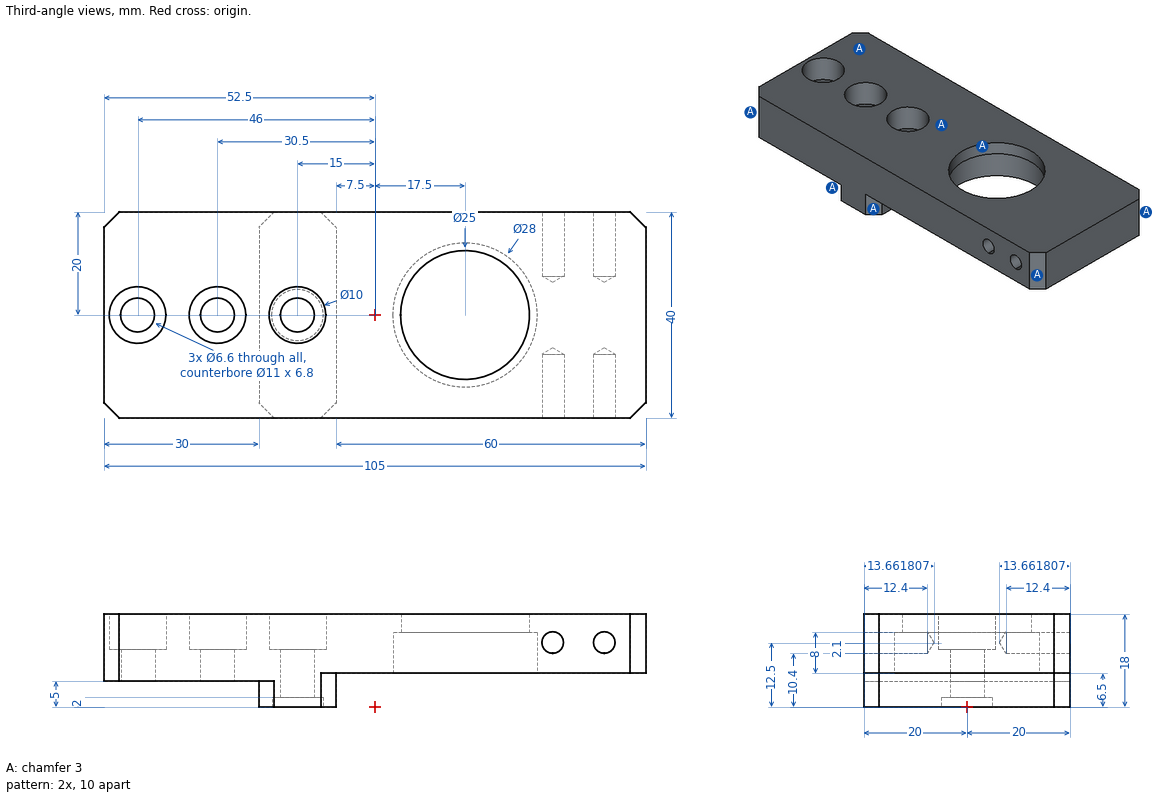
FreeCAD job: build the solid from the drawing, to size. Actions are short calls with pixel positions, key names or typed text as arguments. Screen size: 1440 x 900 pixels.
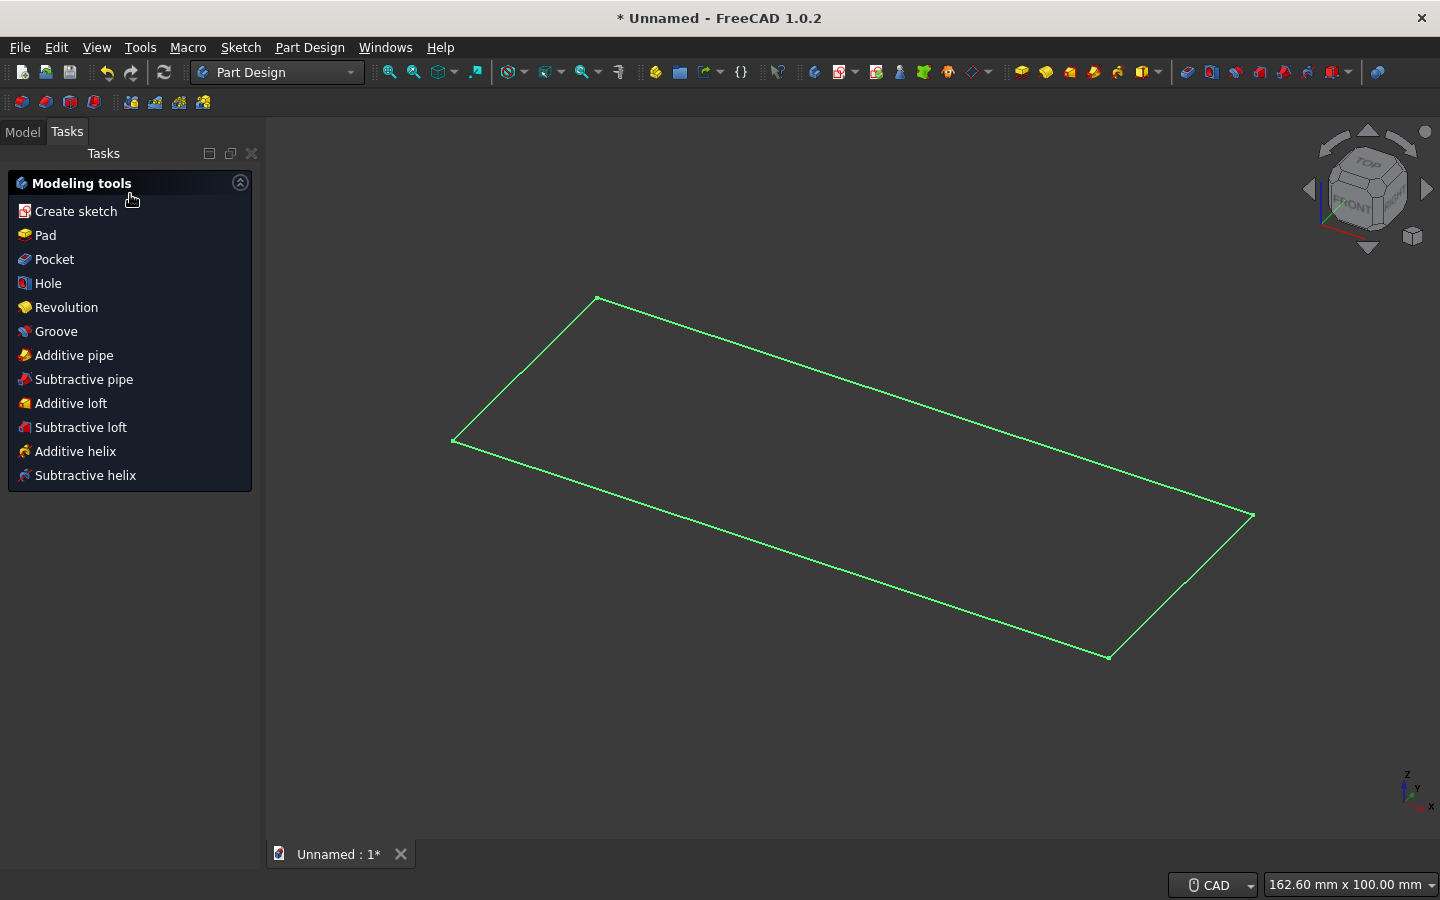
click(1022, 72)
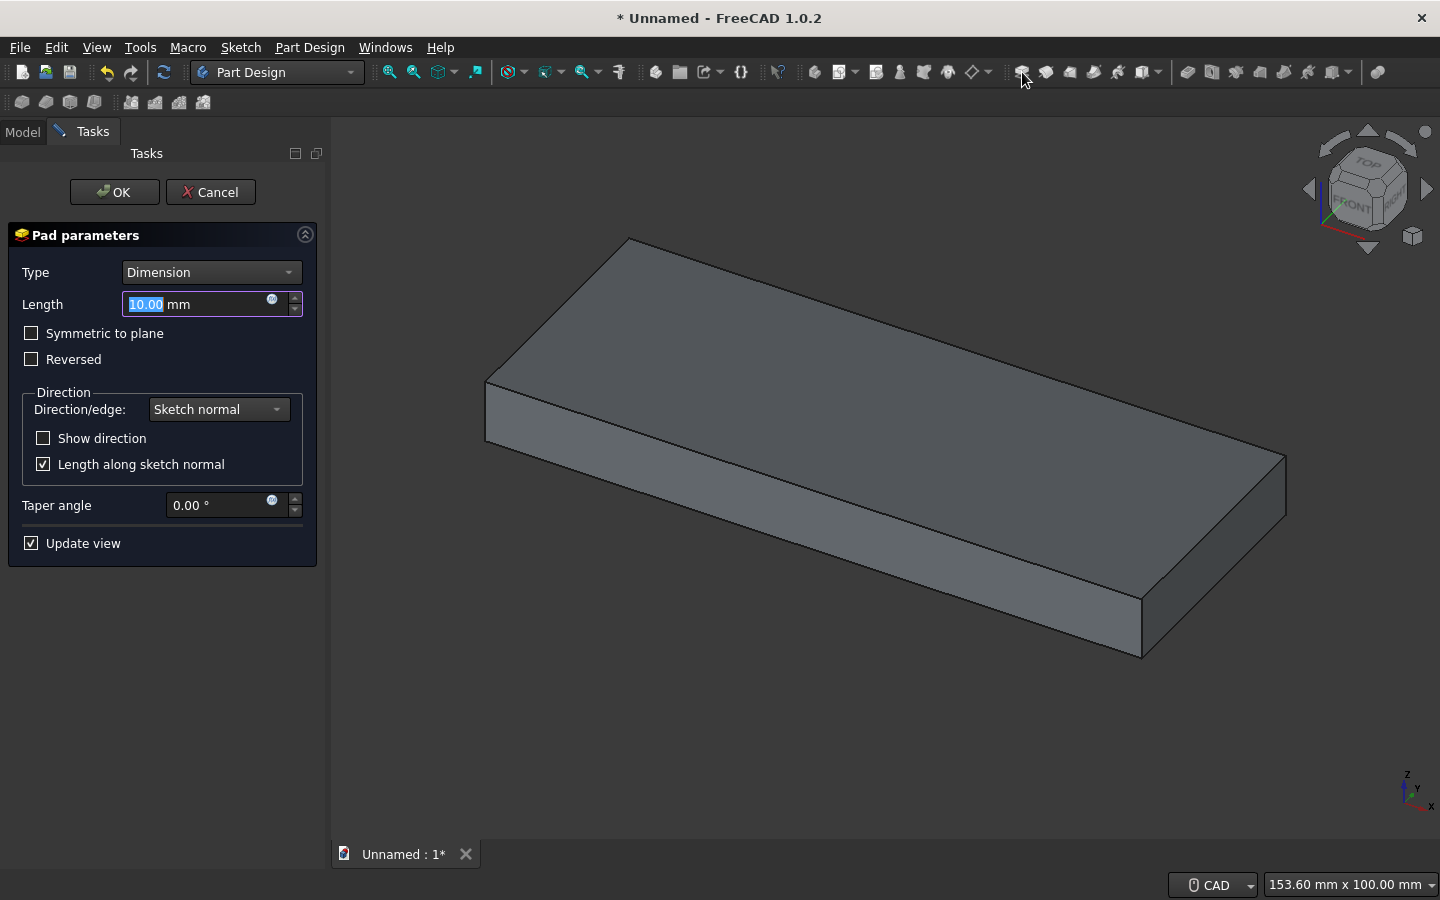
text(18)
key(Tab)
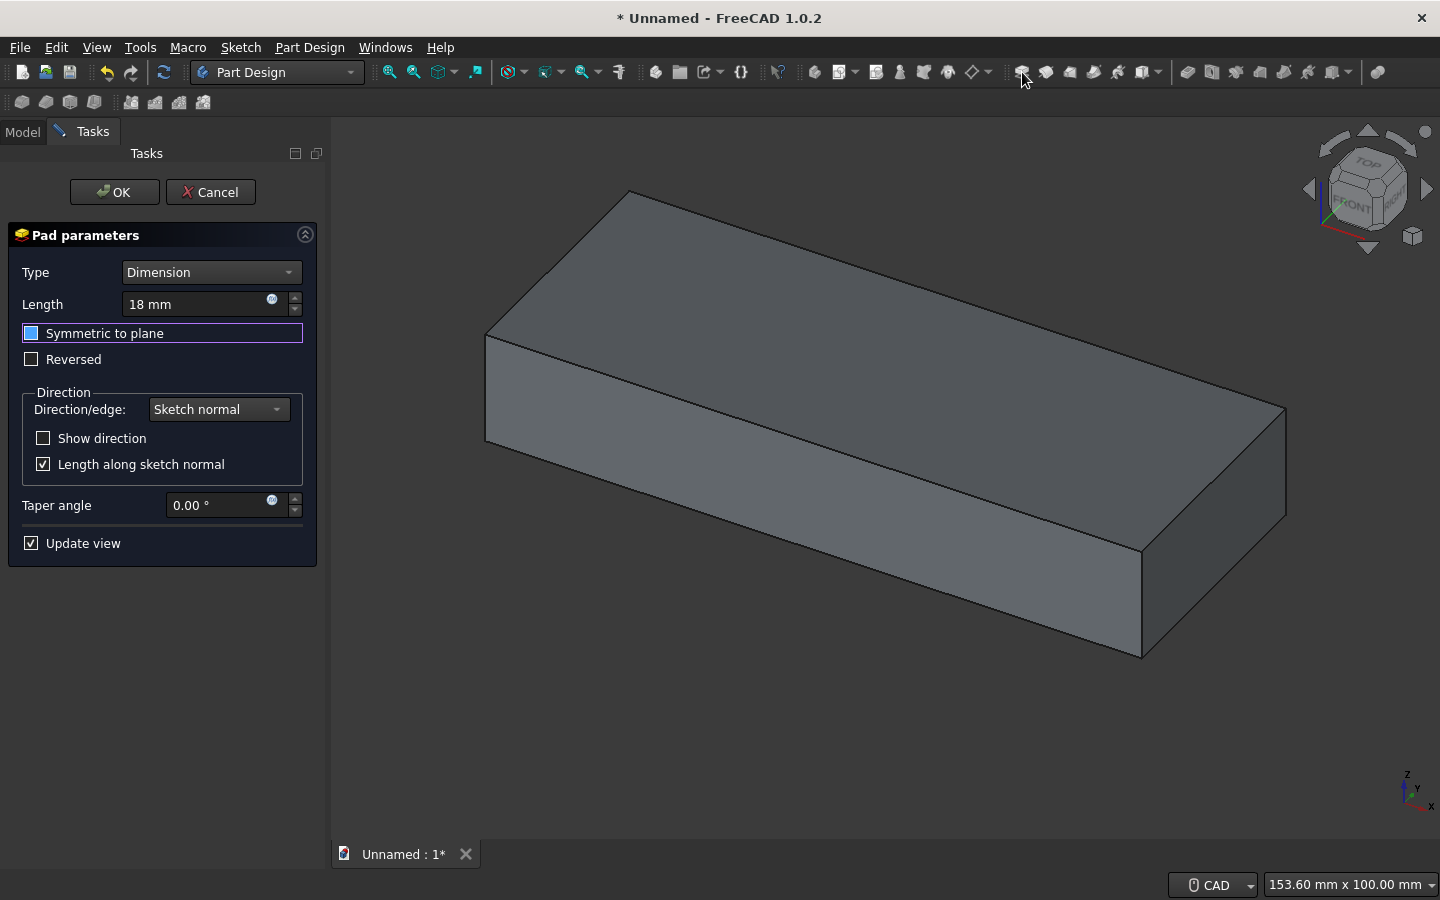
click(115, 192)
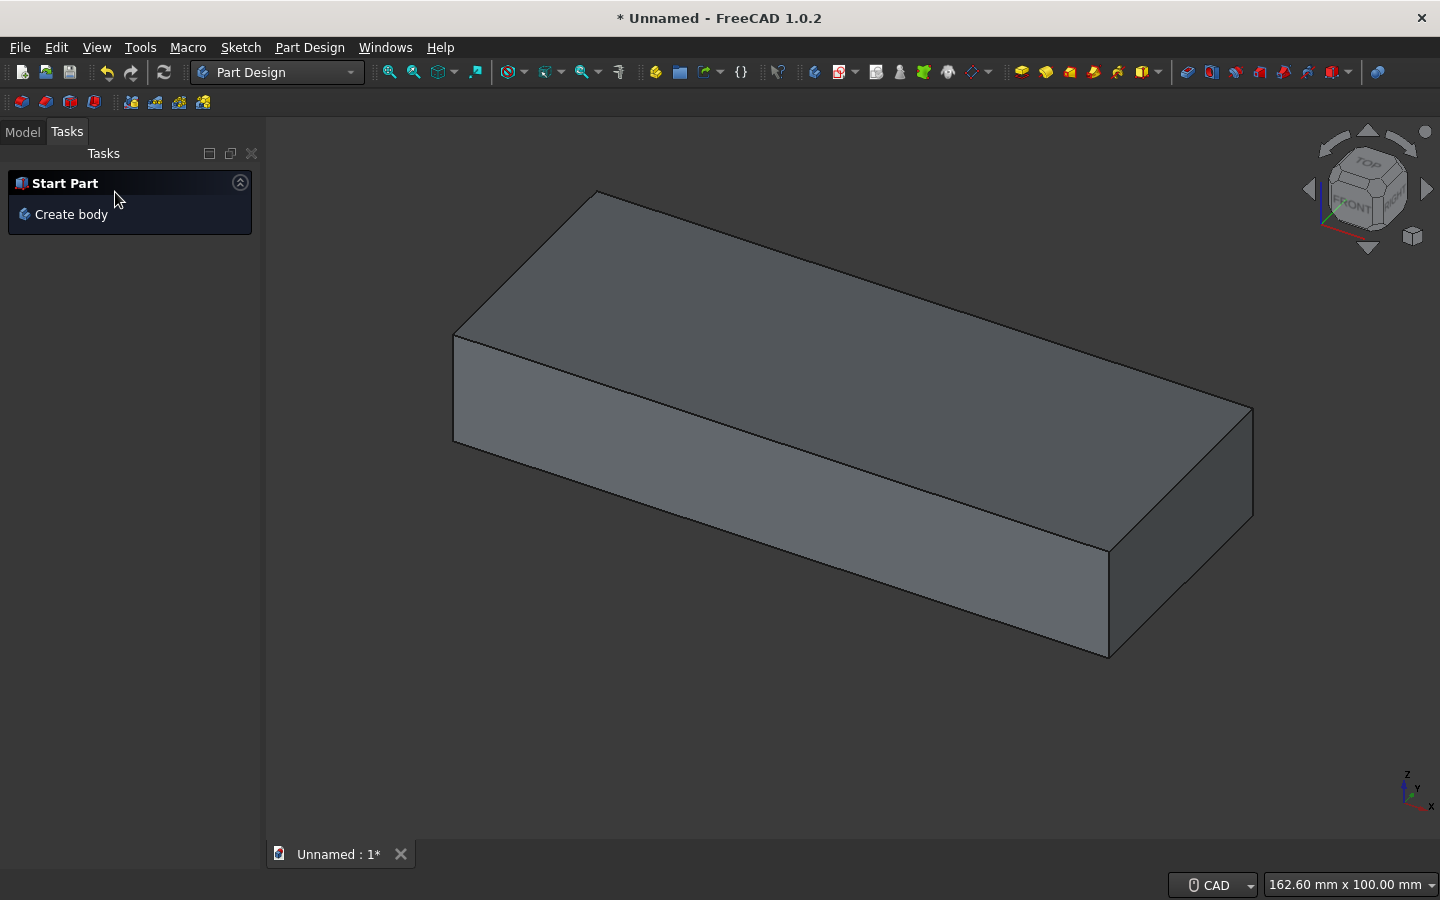
click(840, 72)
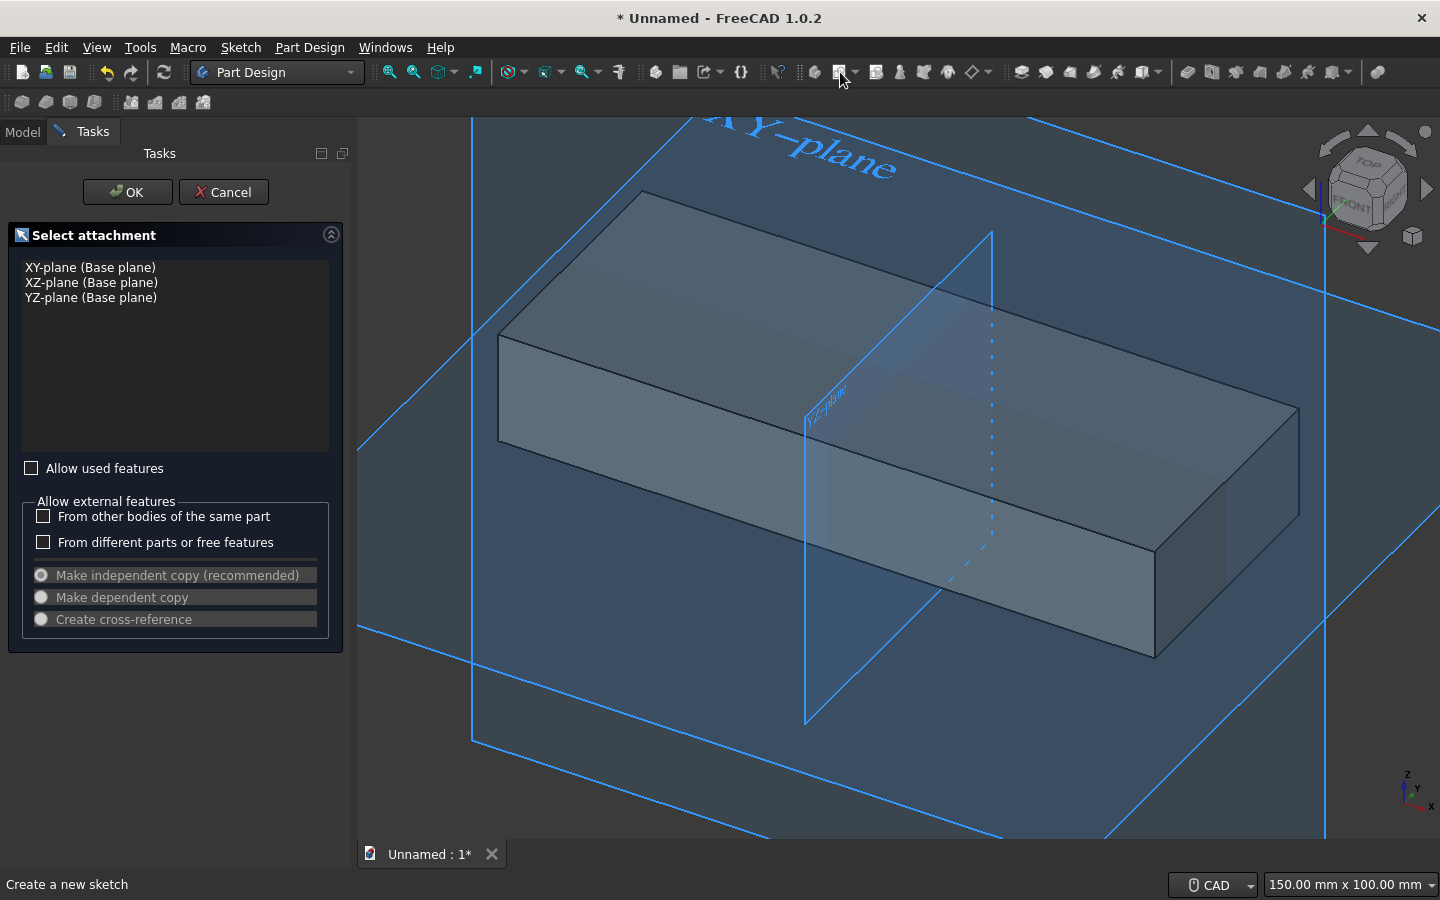
click(82, 268)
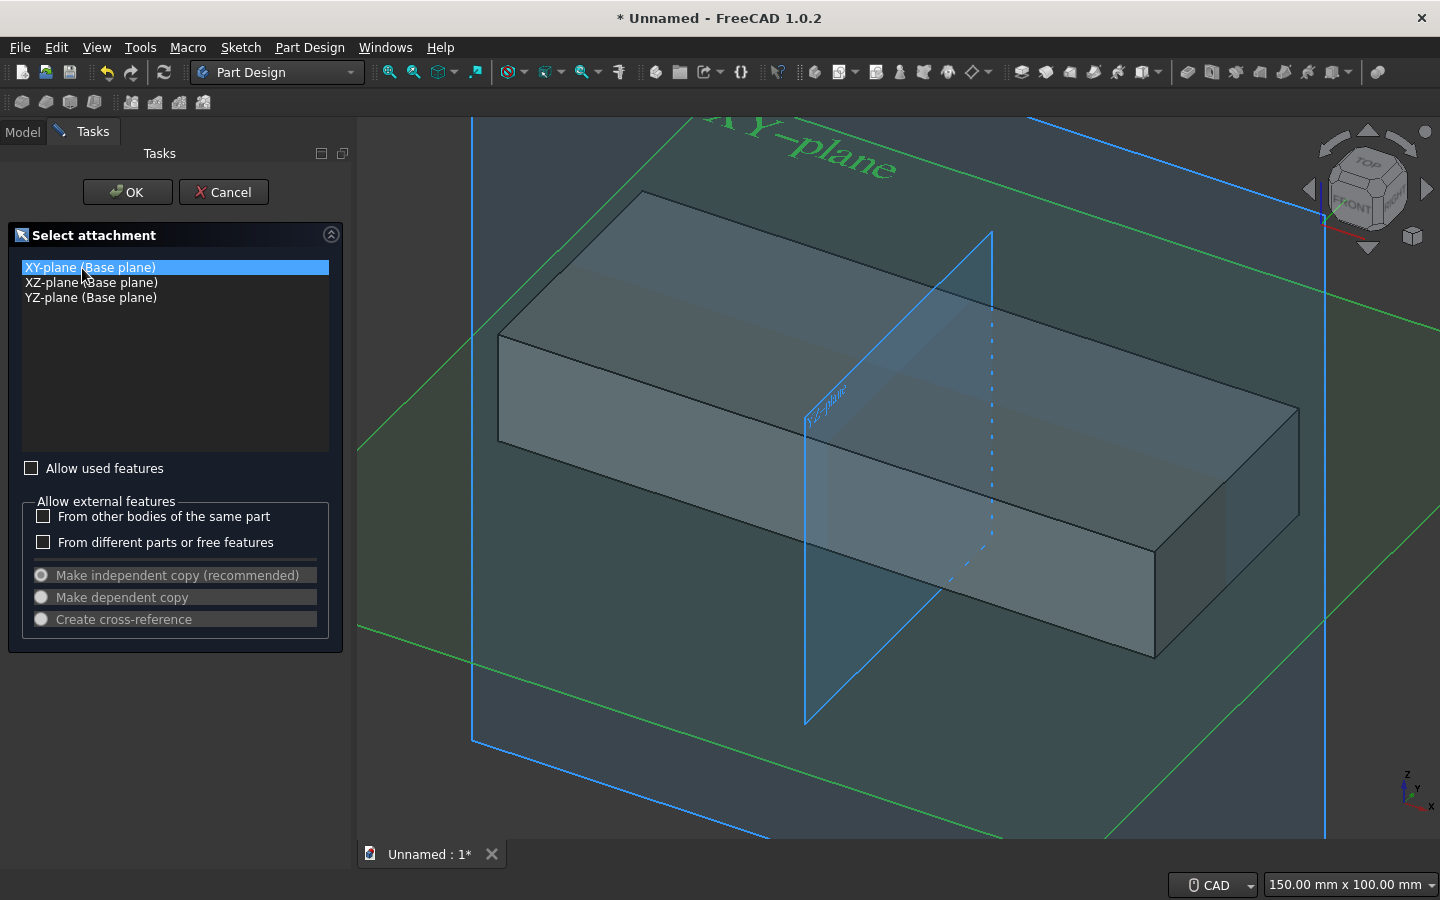
click(128, 192)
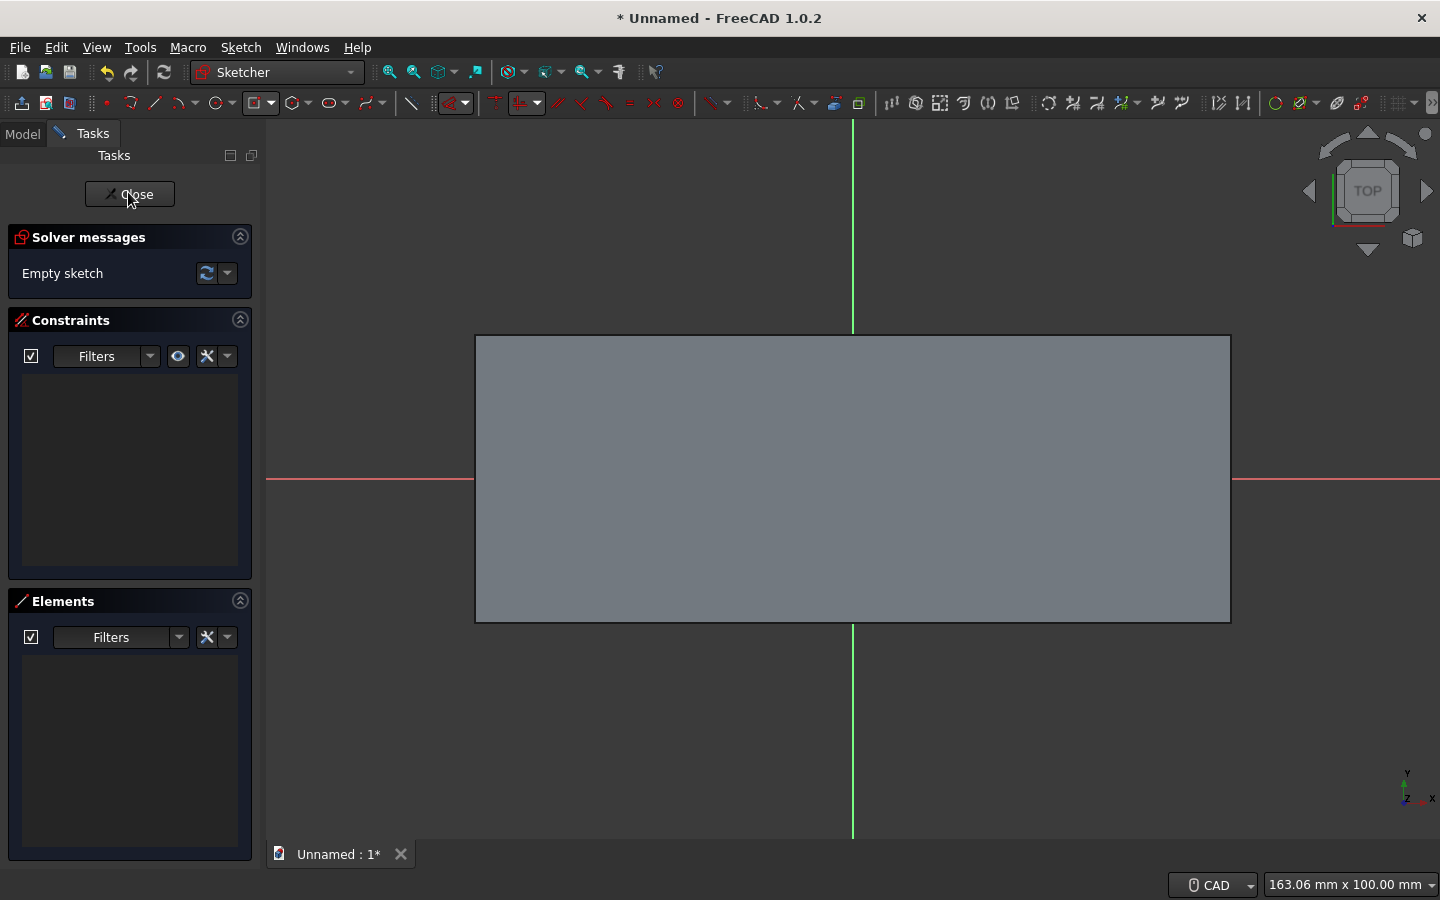
click(70, 104)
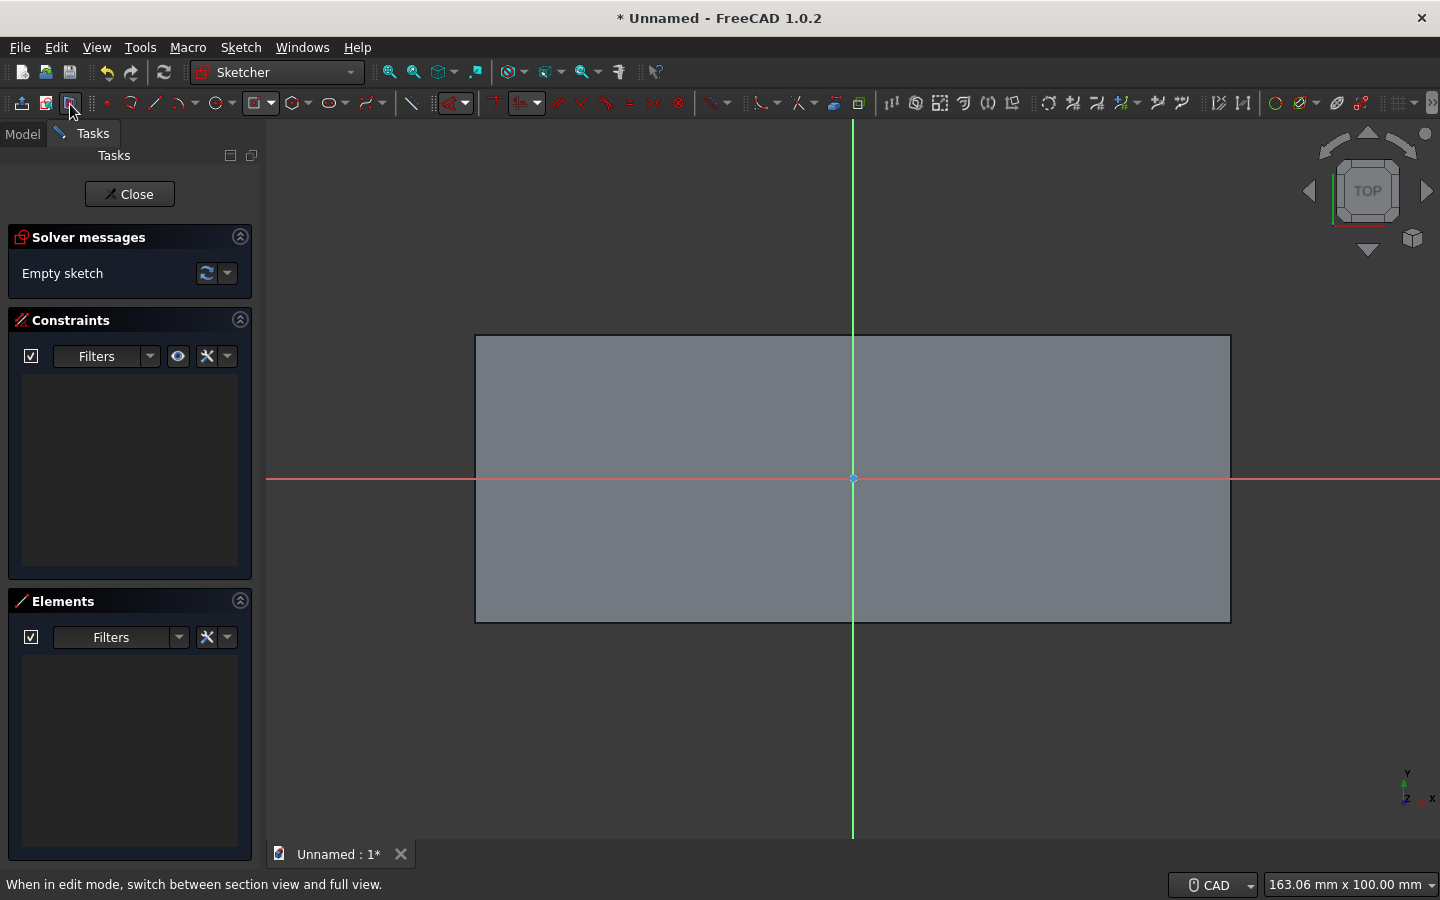
scroll(419, 479, up, 2)